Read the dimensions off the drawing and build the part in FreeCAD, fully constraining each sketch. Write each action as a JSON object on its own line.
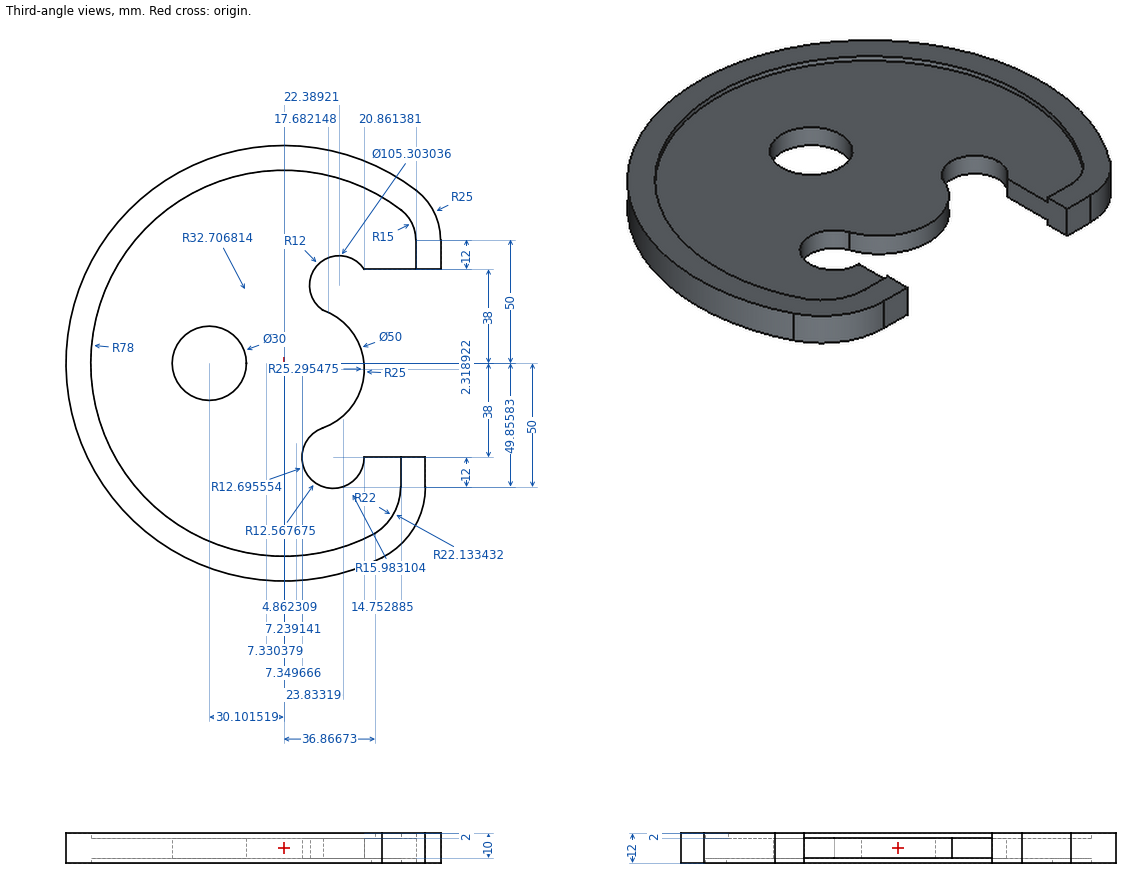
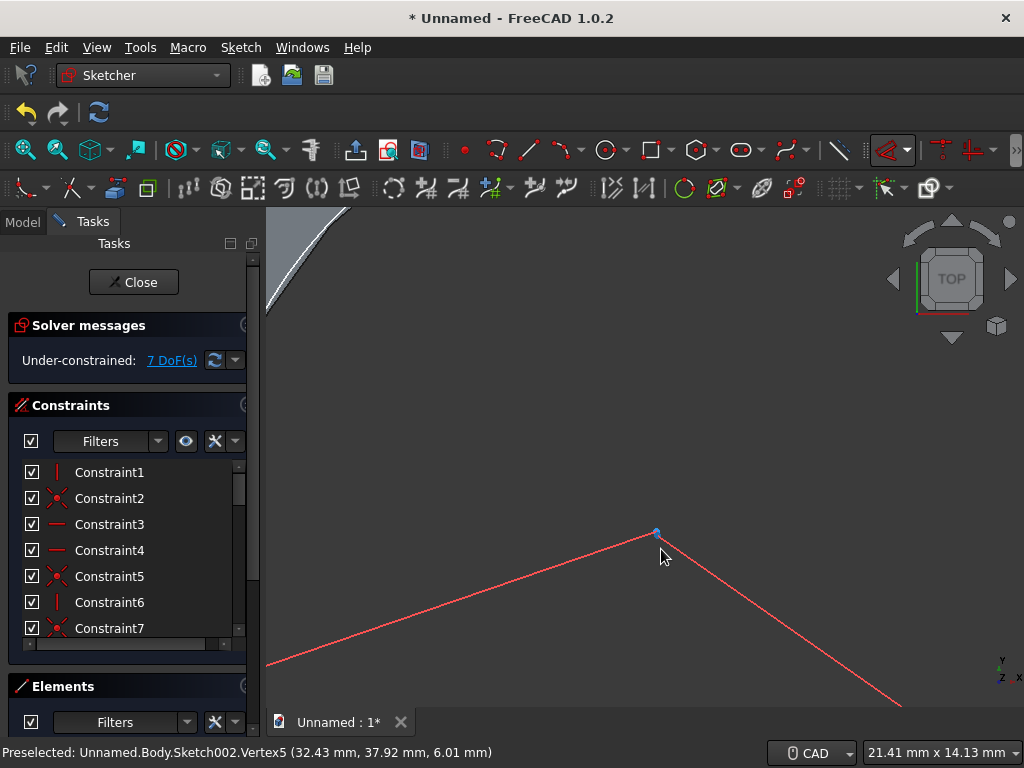
{"action": "left_click", "coordinate": [658, 536]}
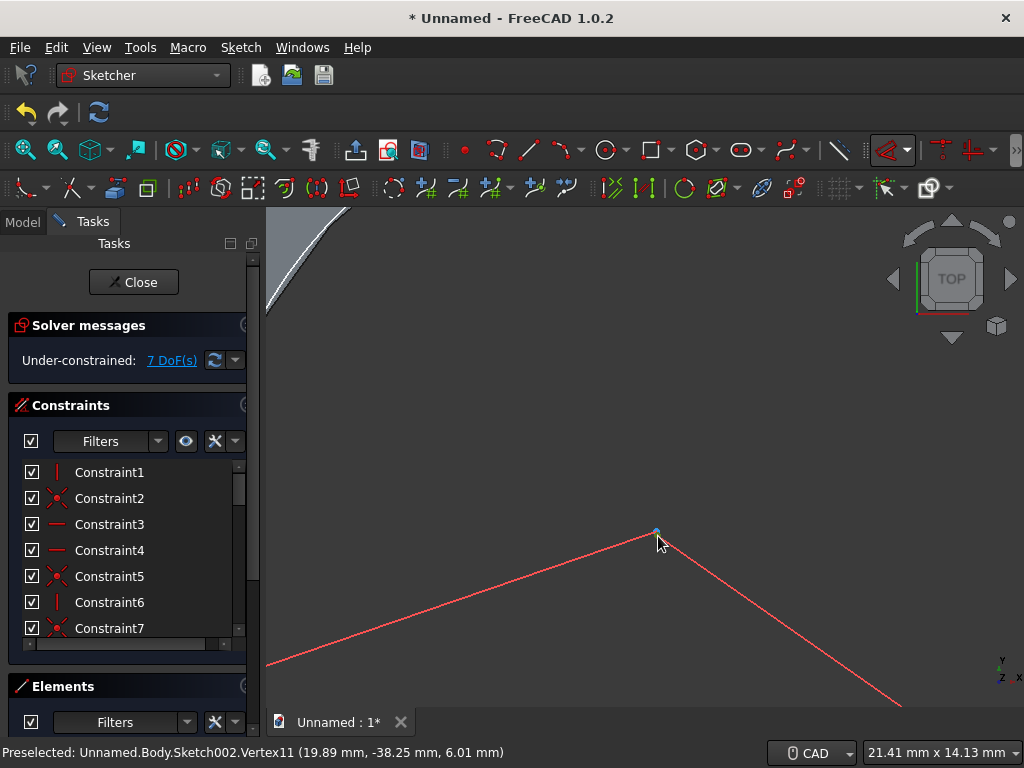
{"action": "key", "text": "i"}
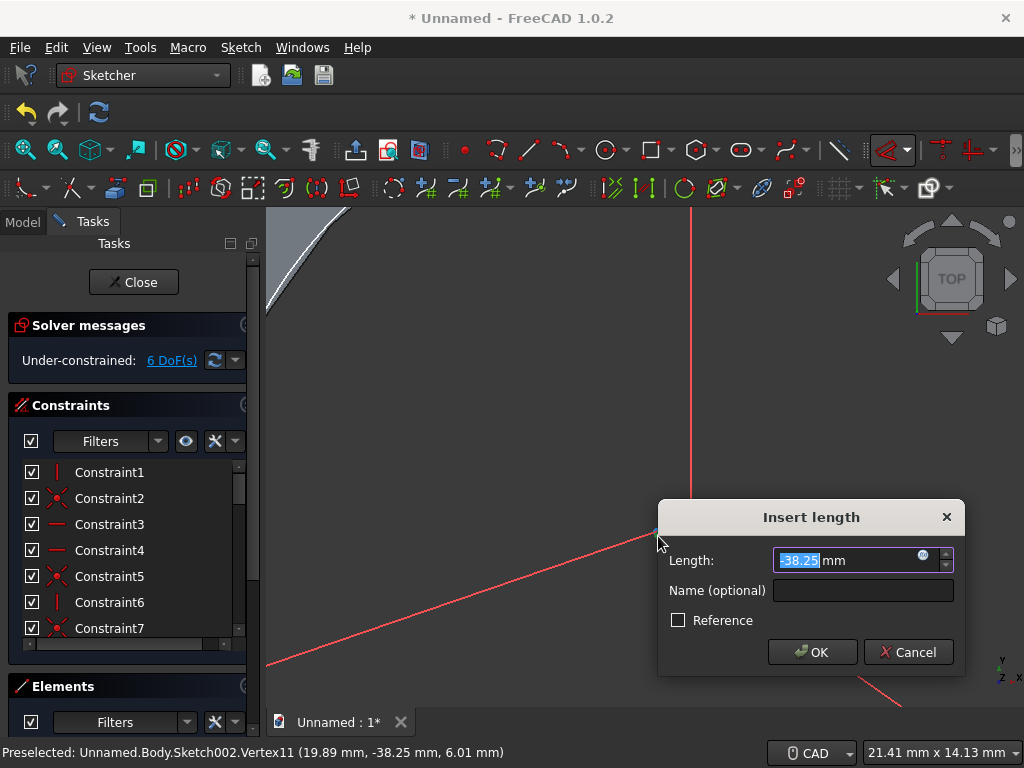
{"action": "type", "text": "-38"}
{"action": "key", "text": "Return"}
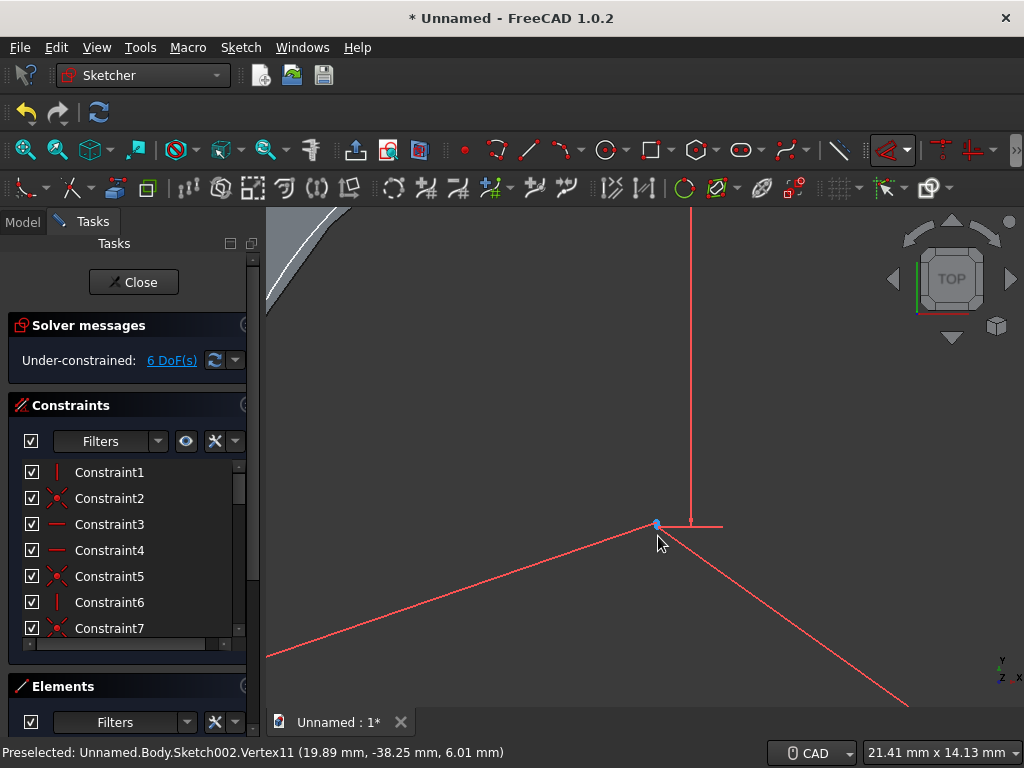
{"action": "scroll", "coordinate": [661, 550], "scroll_direction": "down", "scroll_amount": 13}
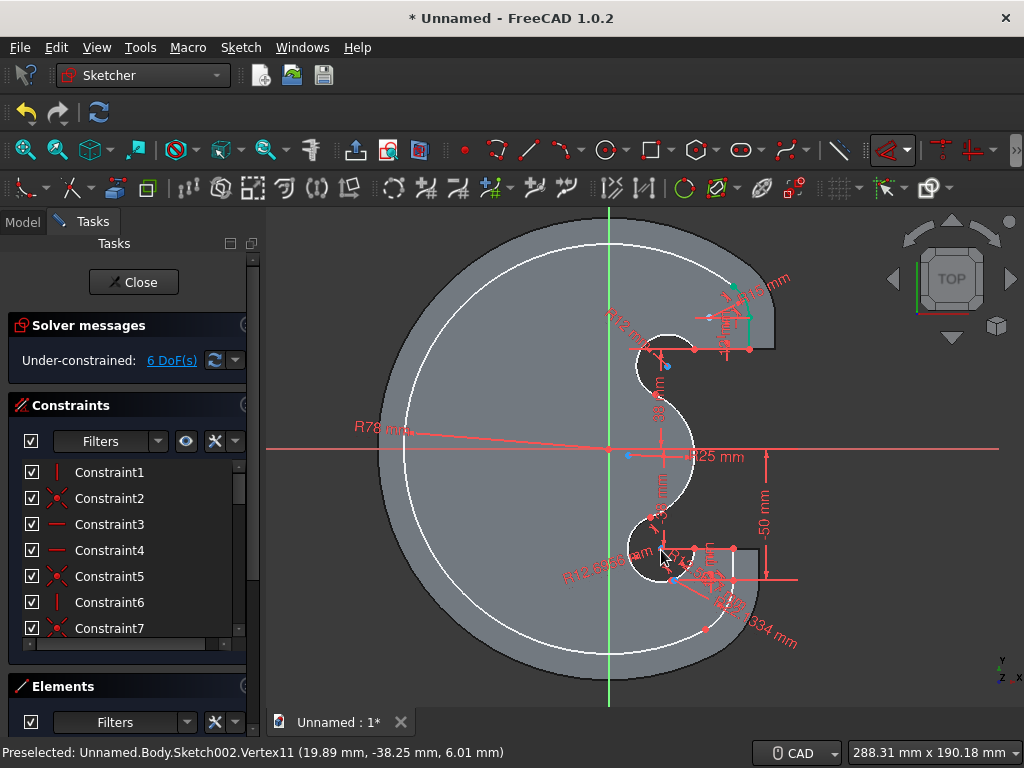
{"action": "left_click", "coordinate": [721, 549]}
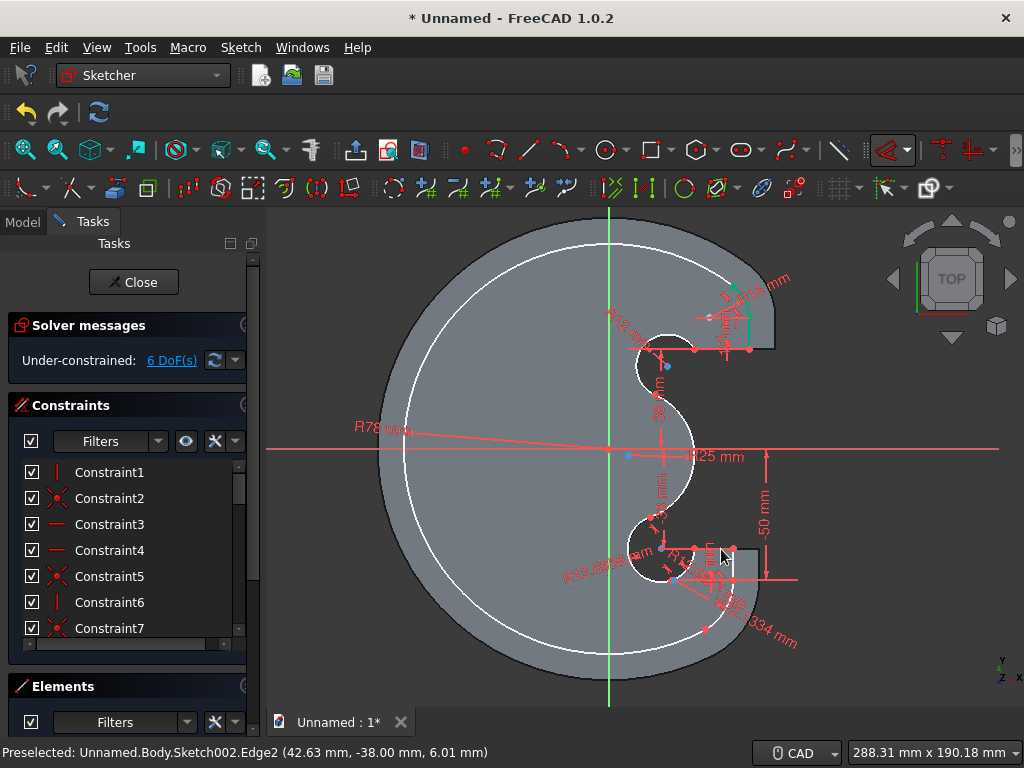
{"action": "key", "text": "l"}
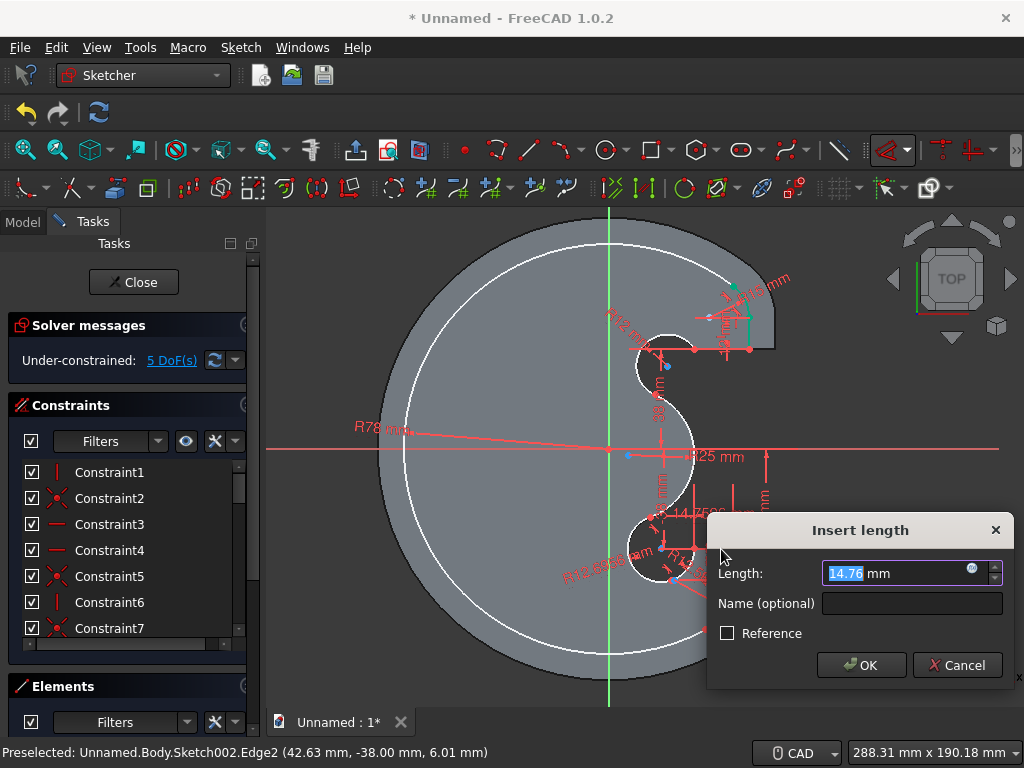
{"action": "type", "text": "14.752885"}
{"action": "key", "text": "Return"}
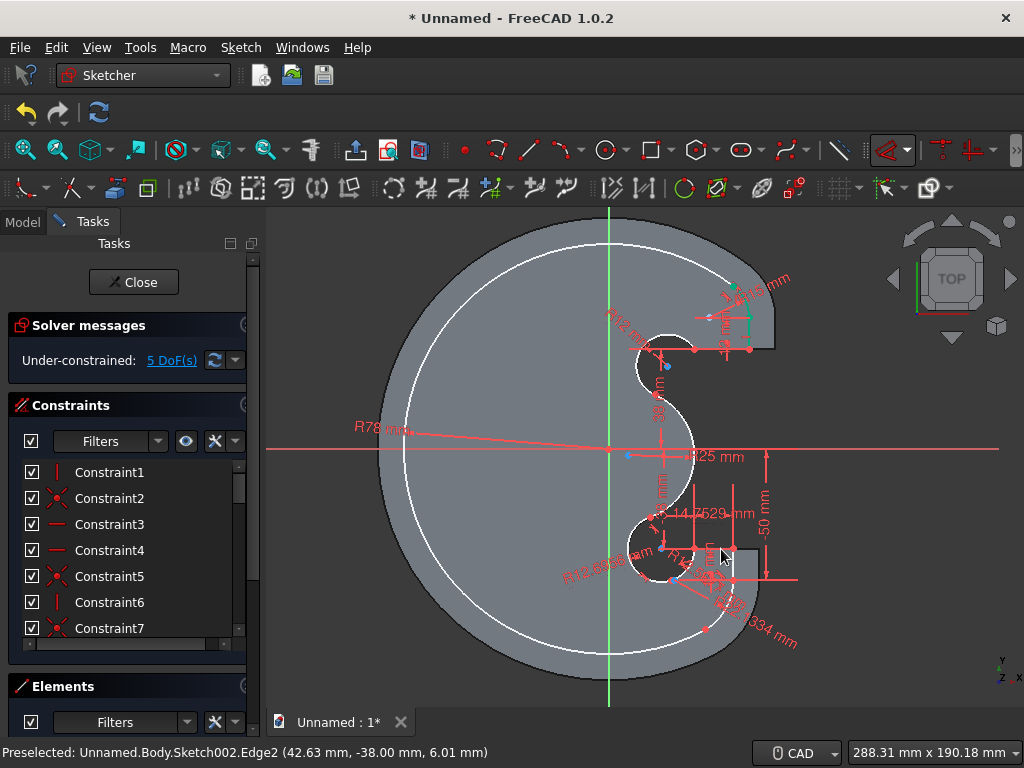
{"action": "left_click", "coordinate": [711, 349]}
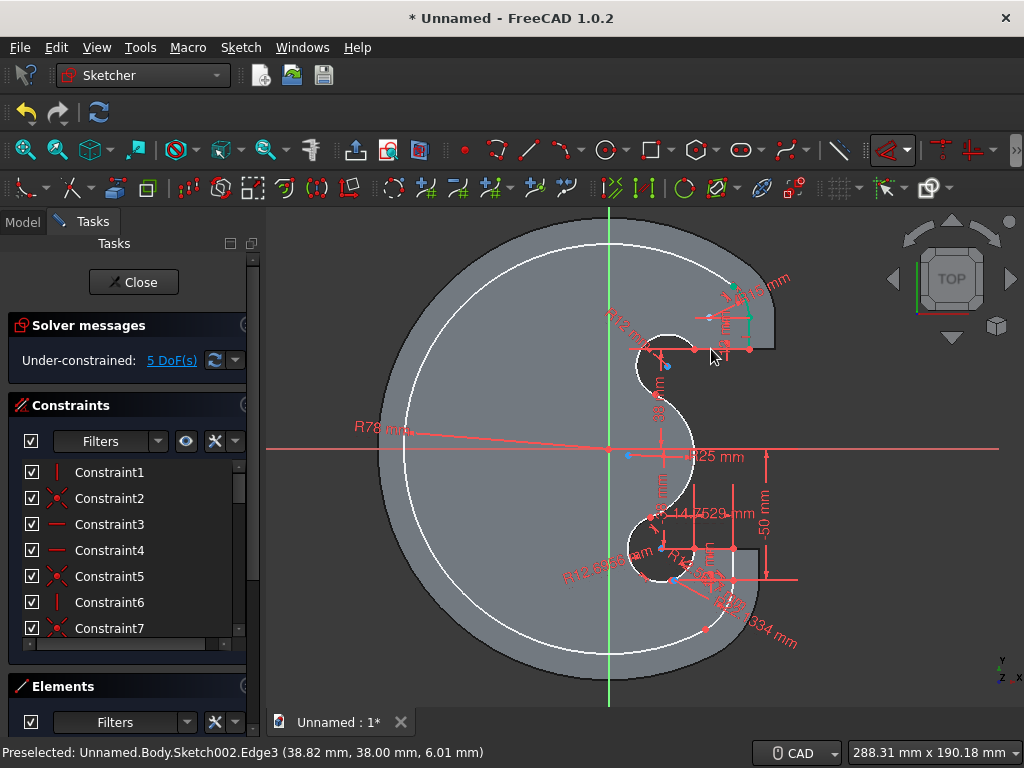
{"action": "left_click", "coordinate": [910, 150]}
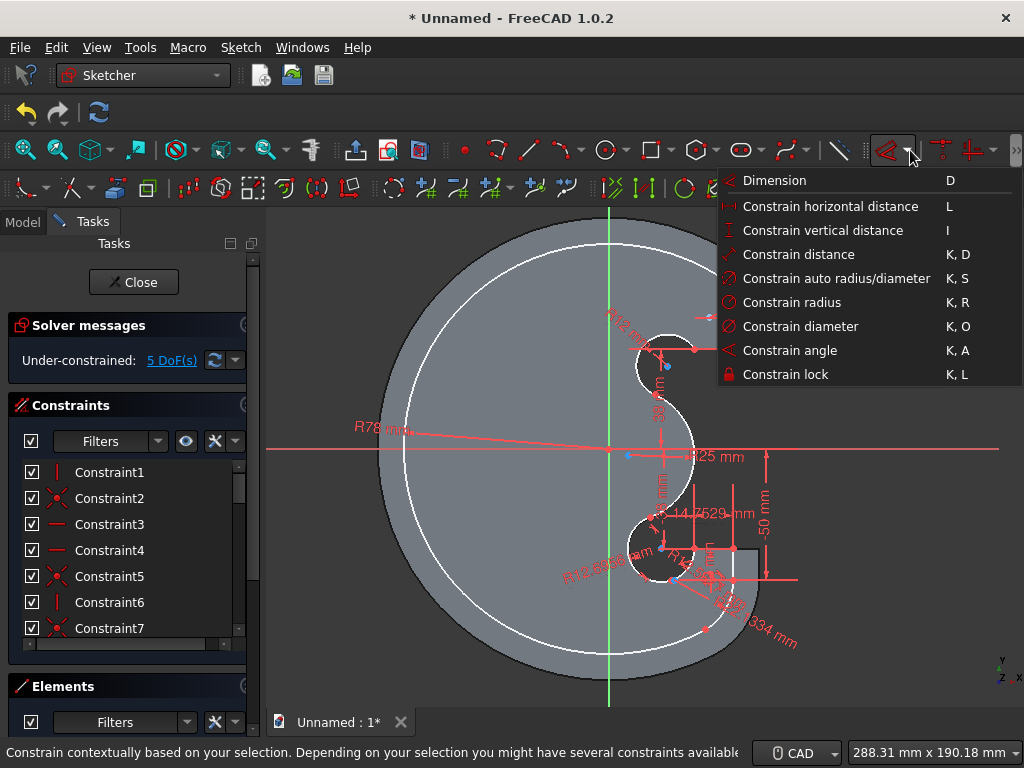
{"action": "left_click", "coordinate": [870, 206]}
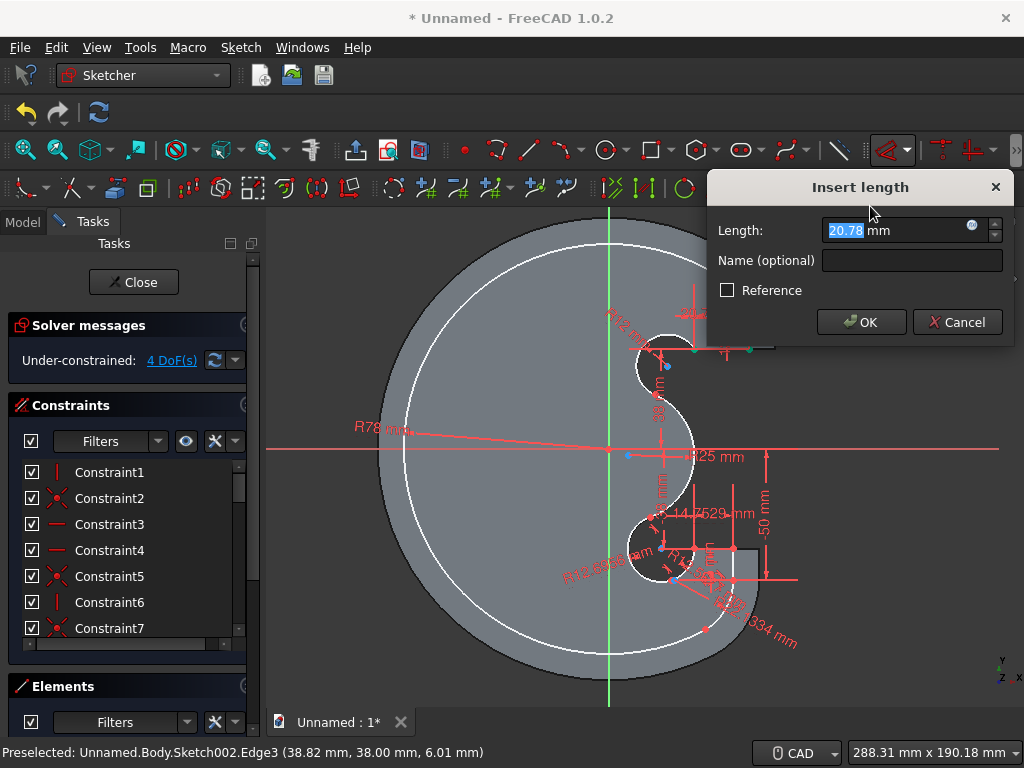
{"action": "type", "text": "20.861381"}
{"action": "key", "text": "Return"}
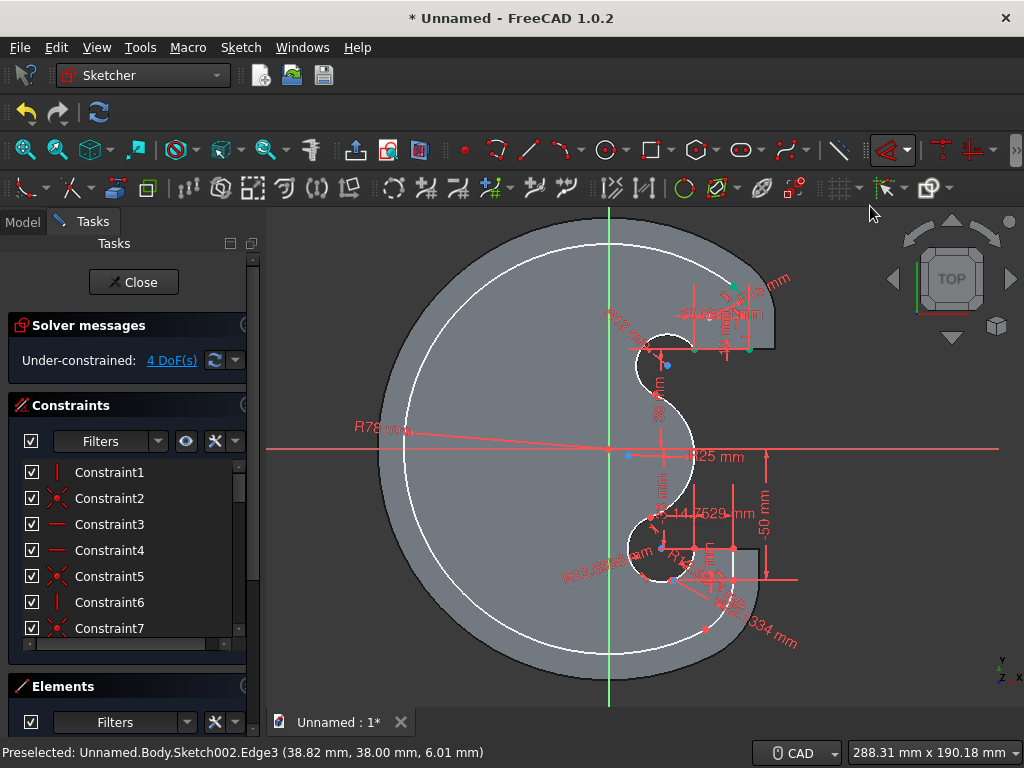
{"action": "scroll", "coordinate": [672, 580], "scroll_direction": "up", "scroll_amount": 7}